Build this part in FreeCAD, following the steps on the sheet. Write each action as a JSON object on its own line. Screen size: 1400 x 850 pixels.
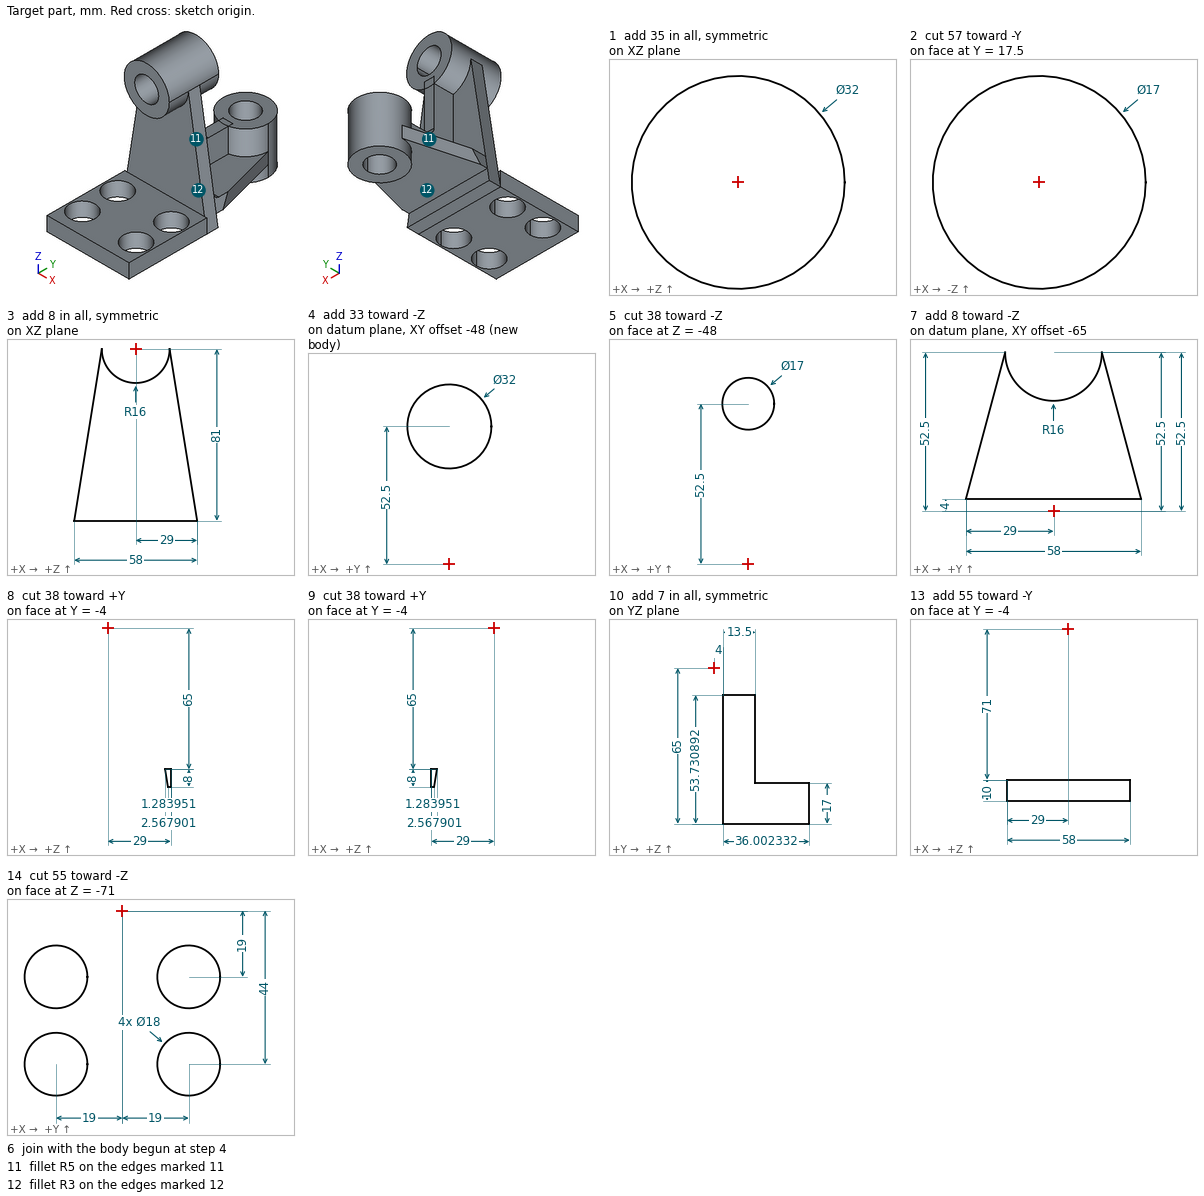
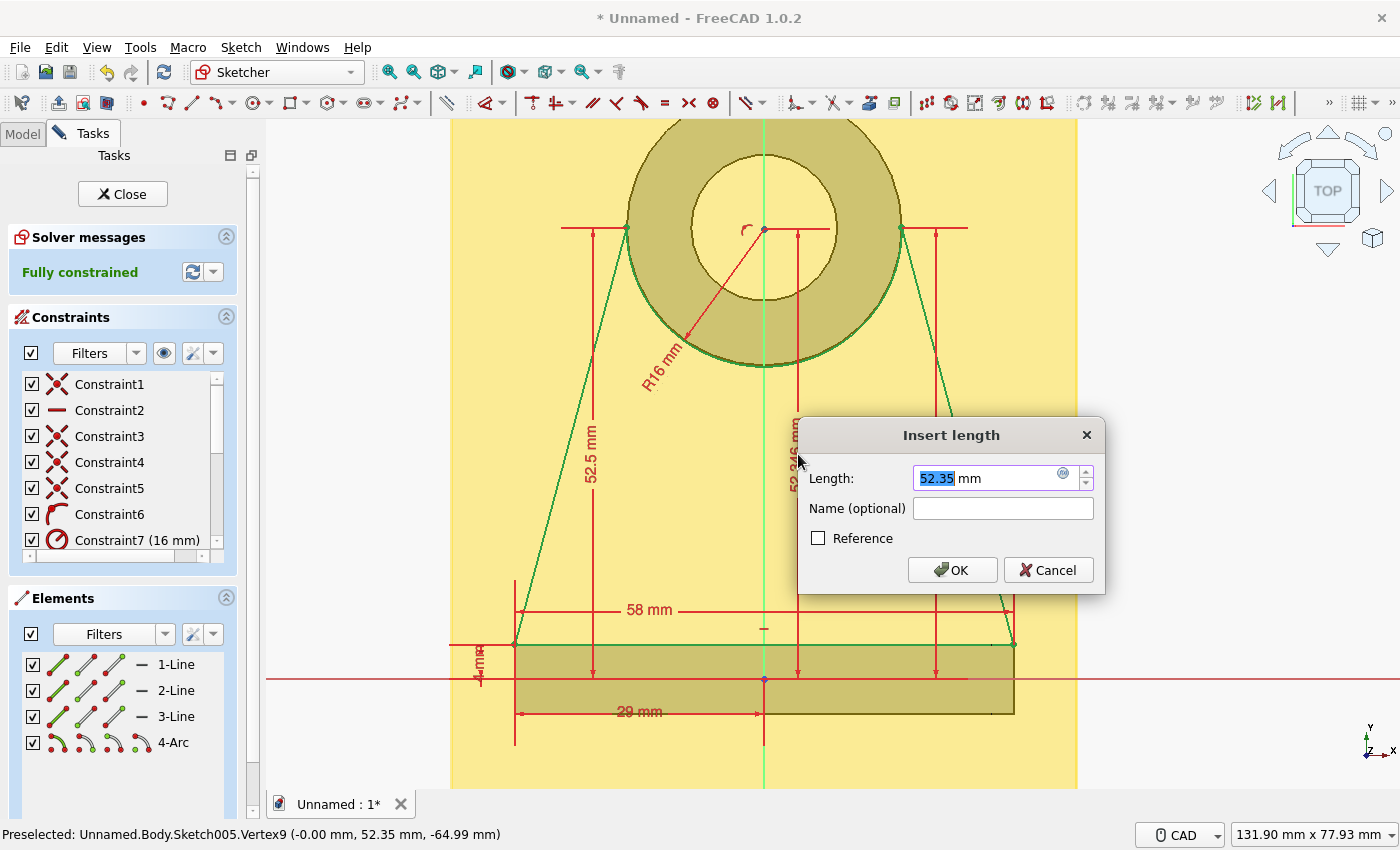
{"action": "type", "text": "52.5"}
{"action": "key", "text": "Return"}
{"action": "key", "text": "Escape"}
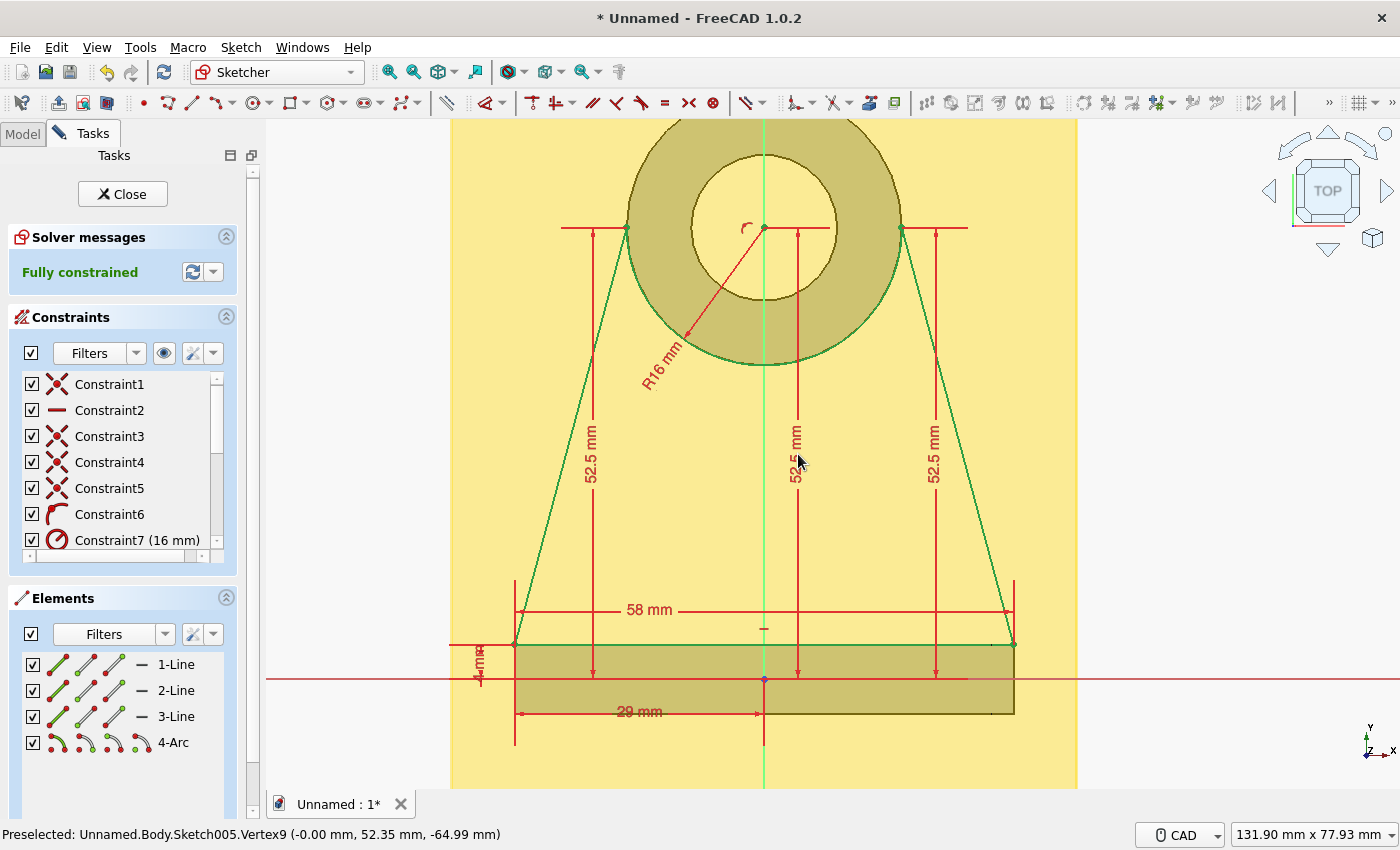
{"action": "left_click", "coordinate": [123, 194]}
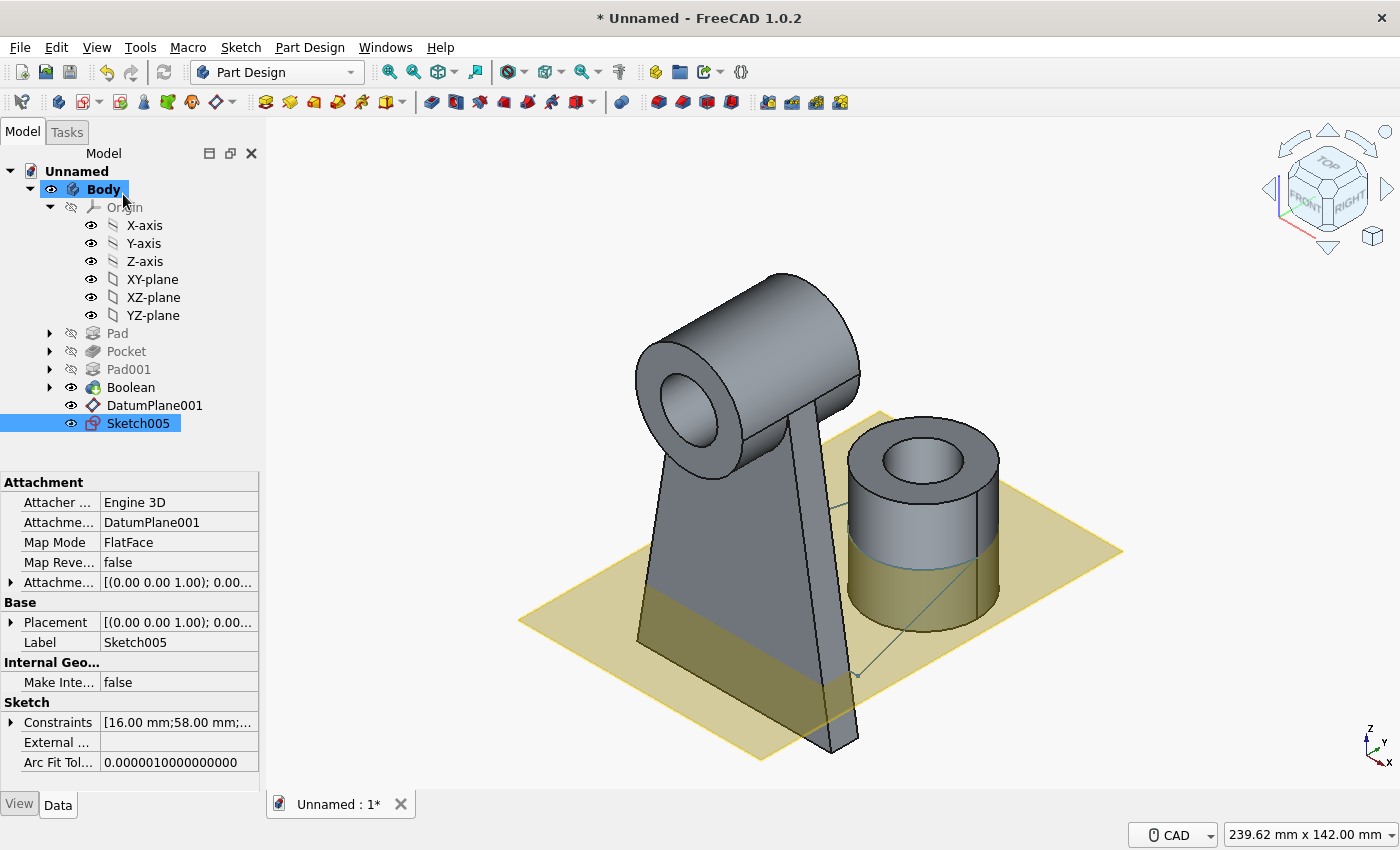
{"action": "left_click", "coordinate": [266, 102]}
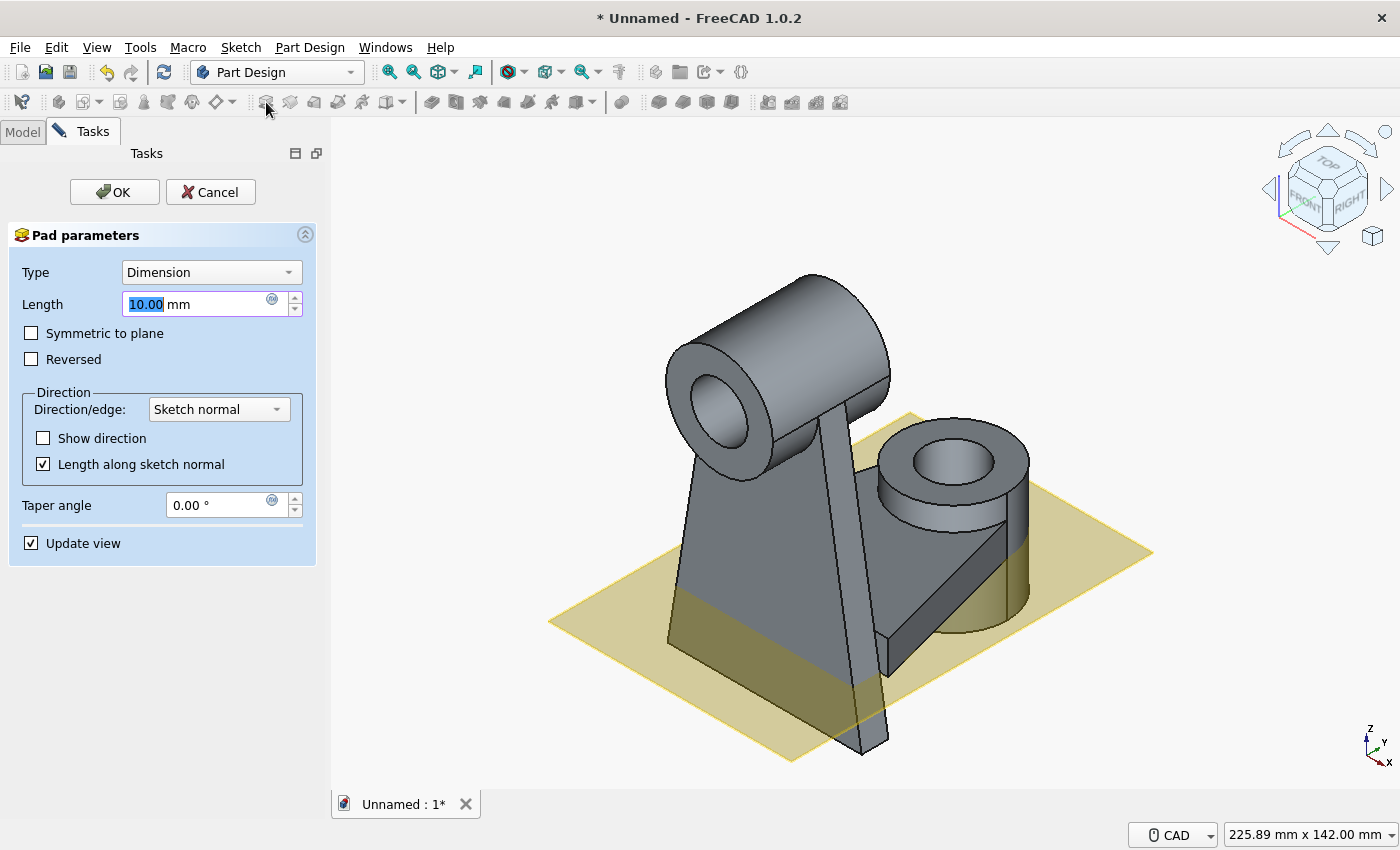
{"action": "type", "text": "8"}
{"action": "key", "text": "Tab"}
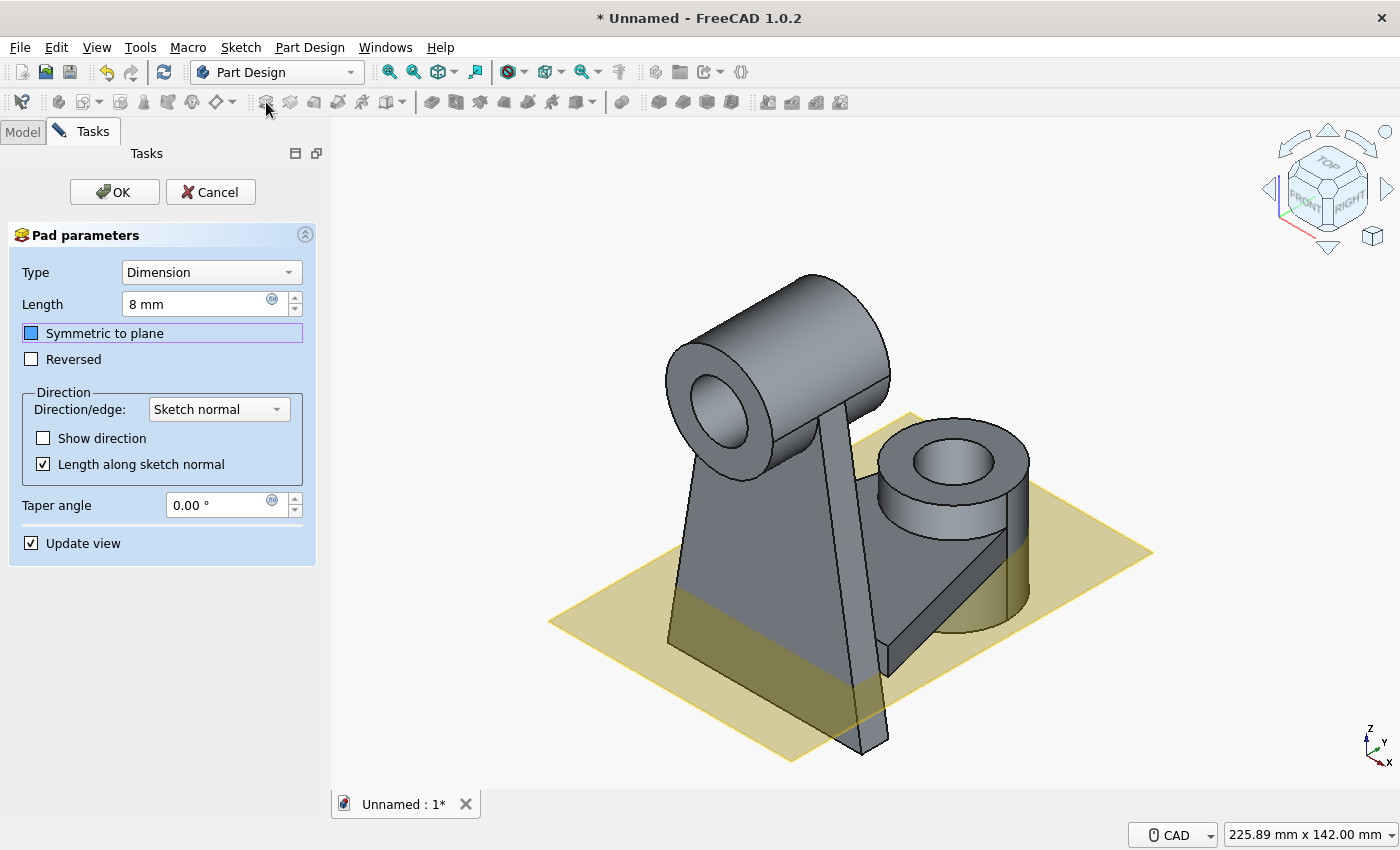
{"action": "left_click", "coordinate": [30, 359]}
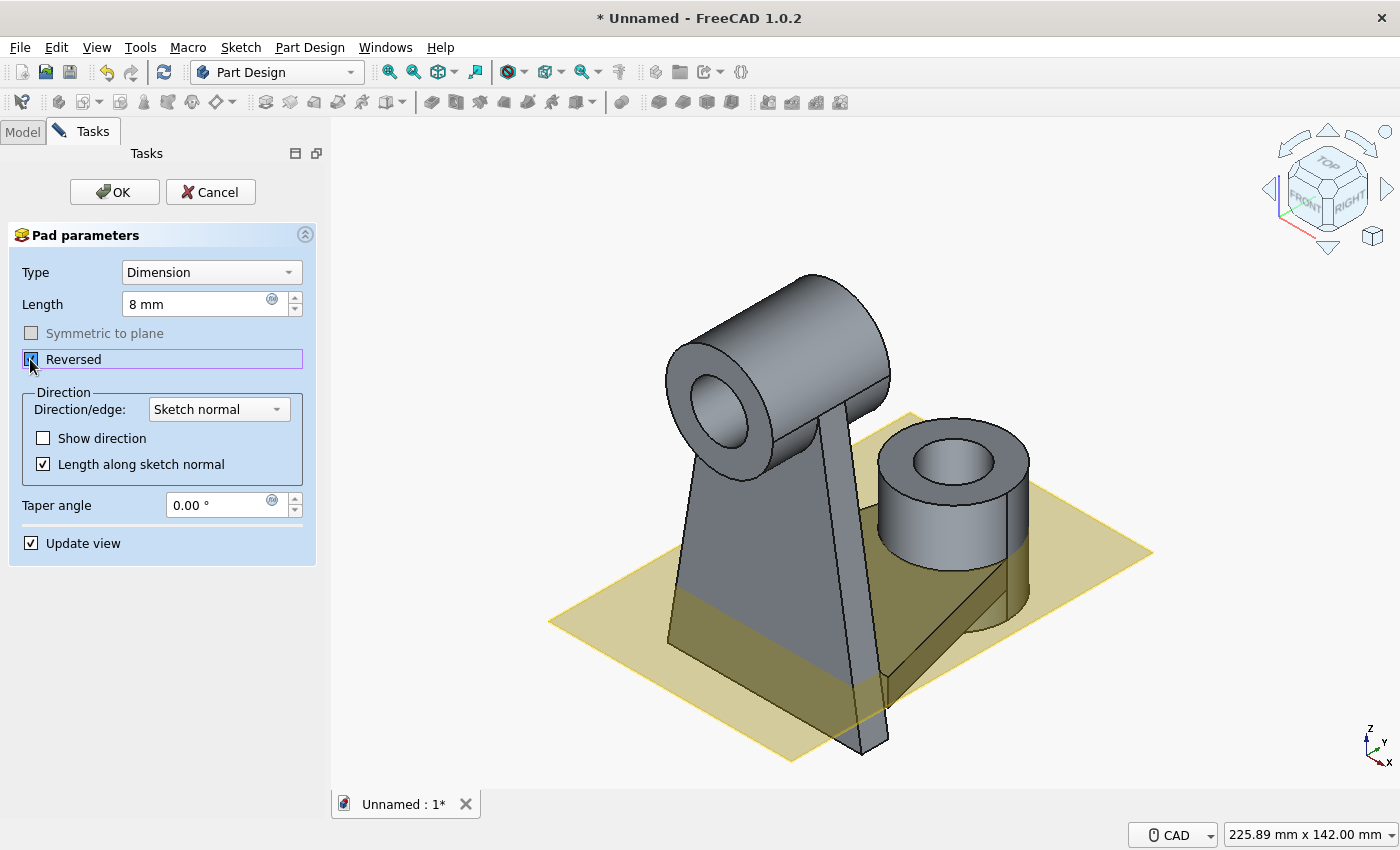
{"action": "left_click", "coordinate": [115, 192]}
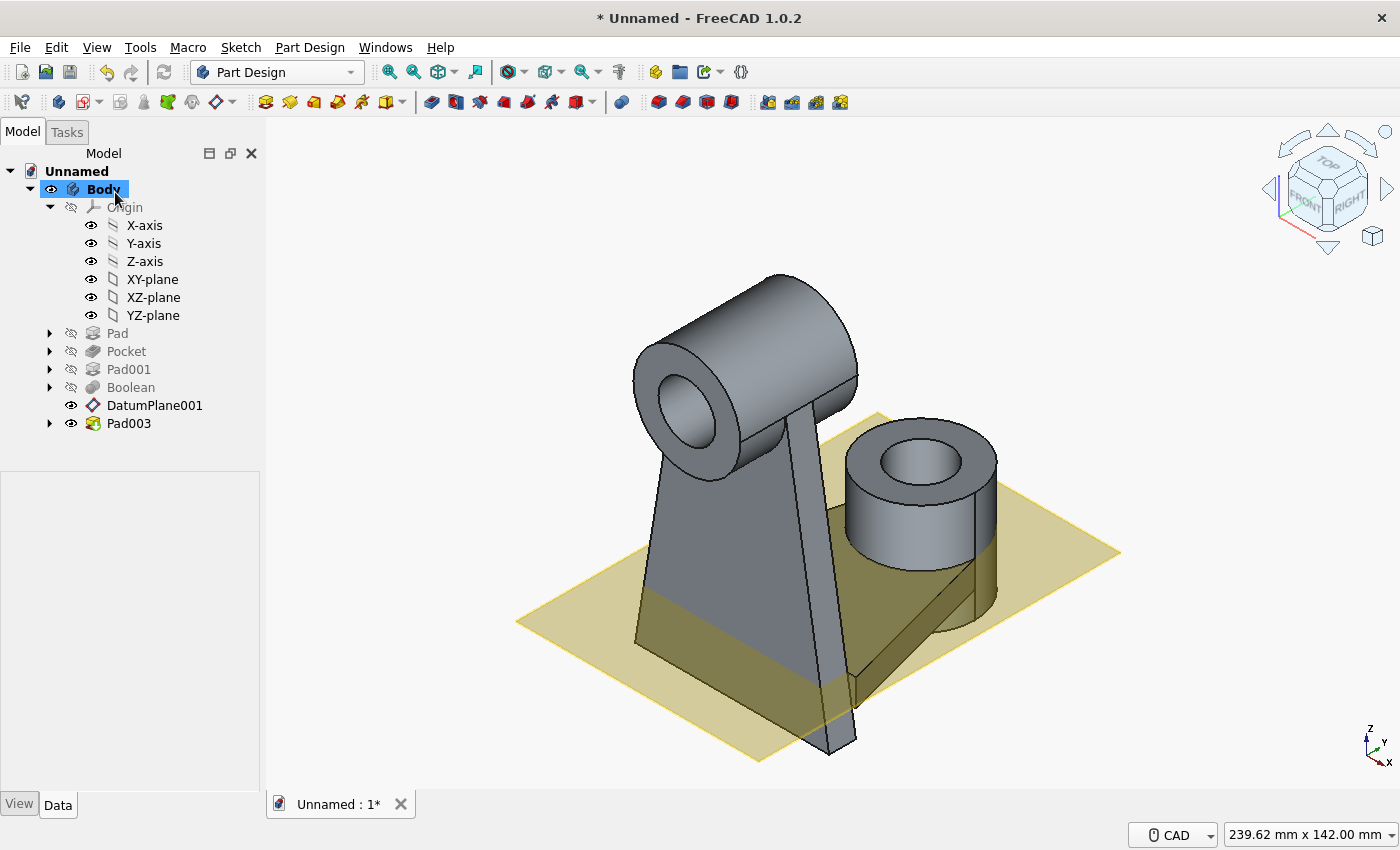
{"action": "left_click", "coordinate": [116, 405]}
{"action": "key", "text": "space"}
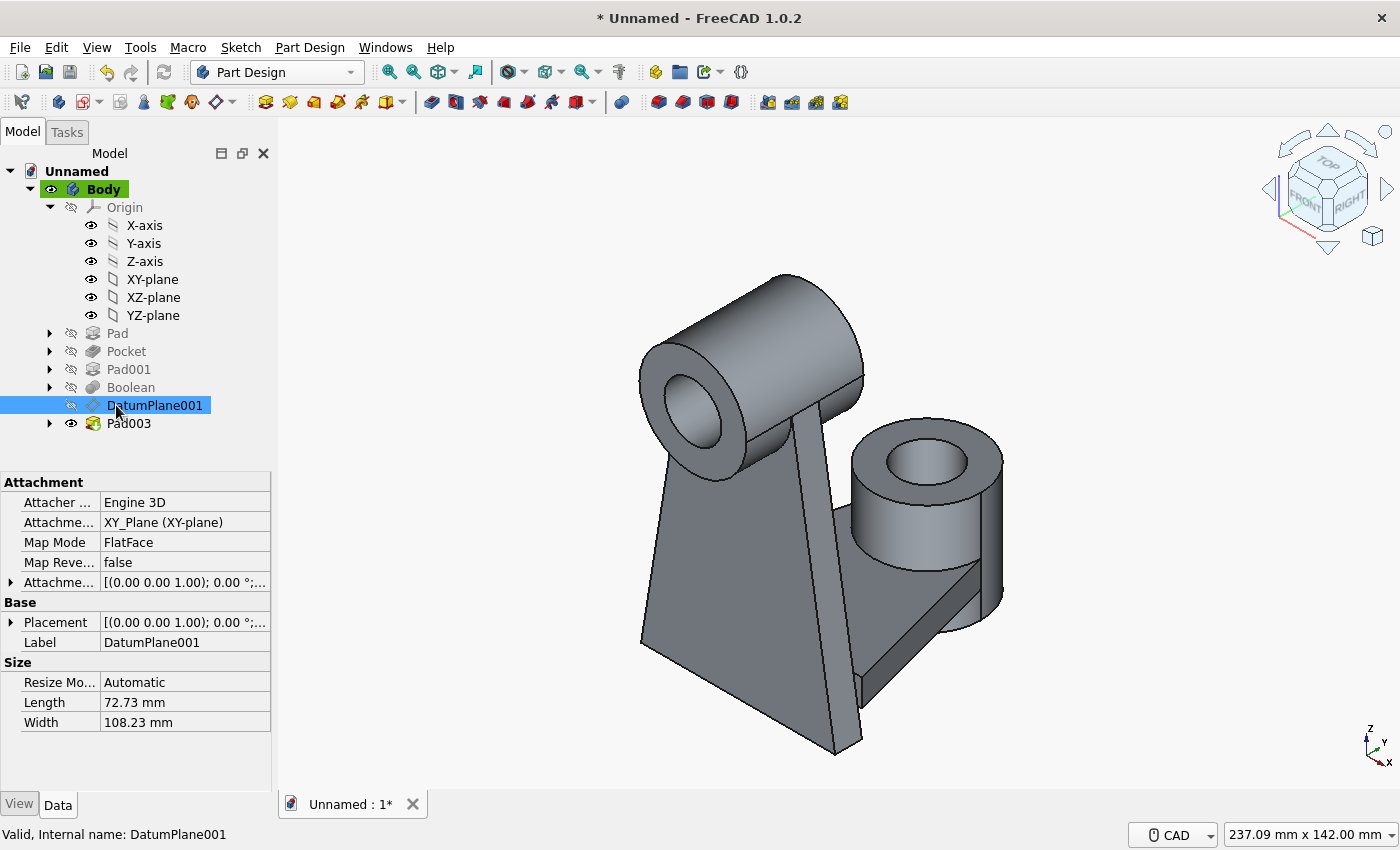
{"action": "left_click", "coordinate": [738, 586]}